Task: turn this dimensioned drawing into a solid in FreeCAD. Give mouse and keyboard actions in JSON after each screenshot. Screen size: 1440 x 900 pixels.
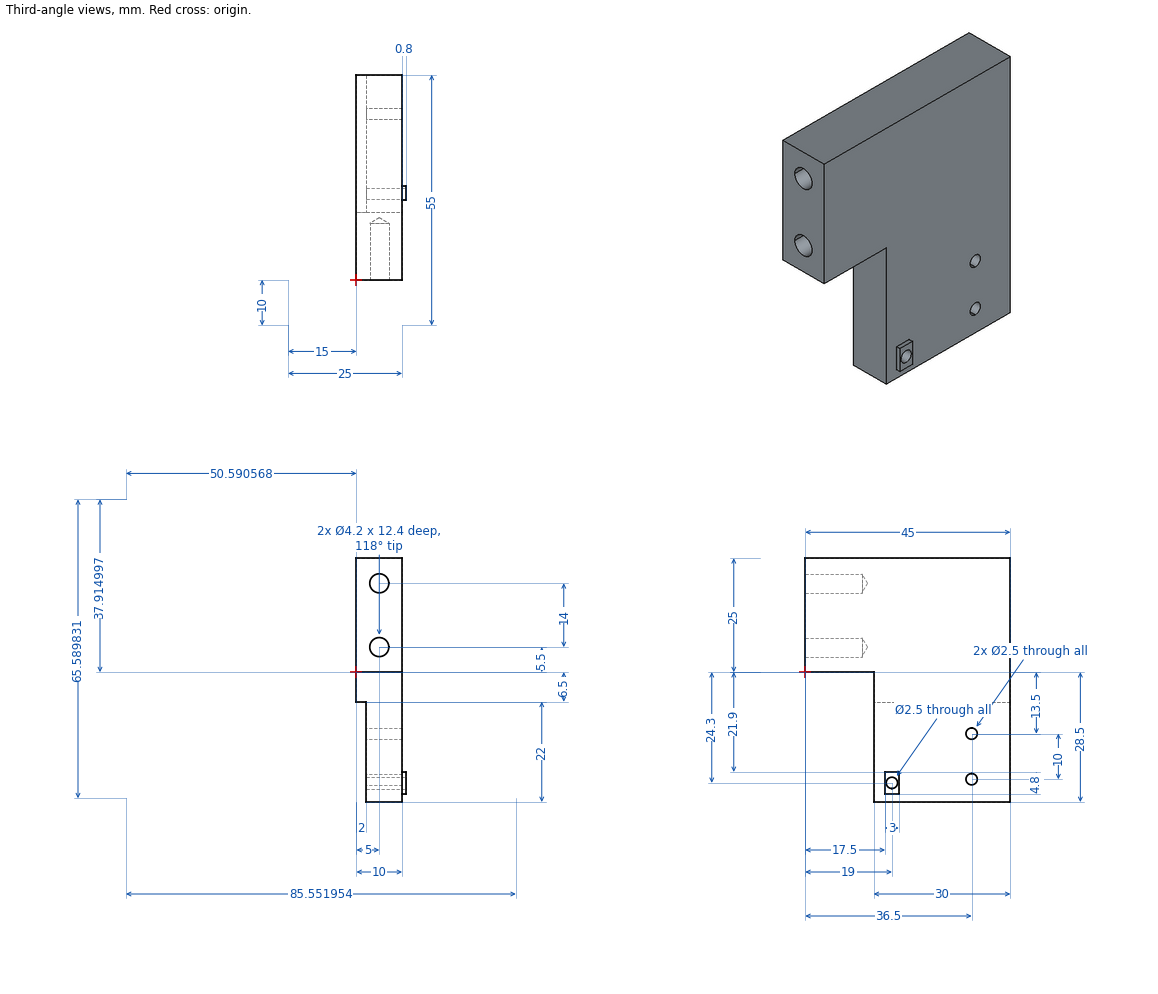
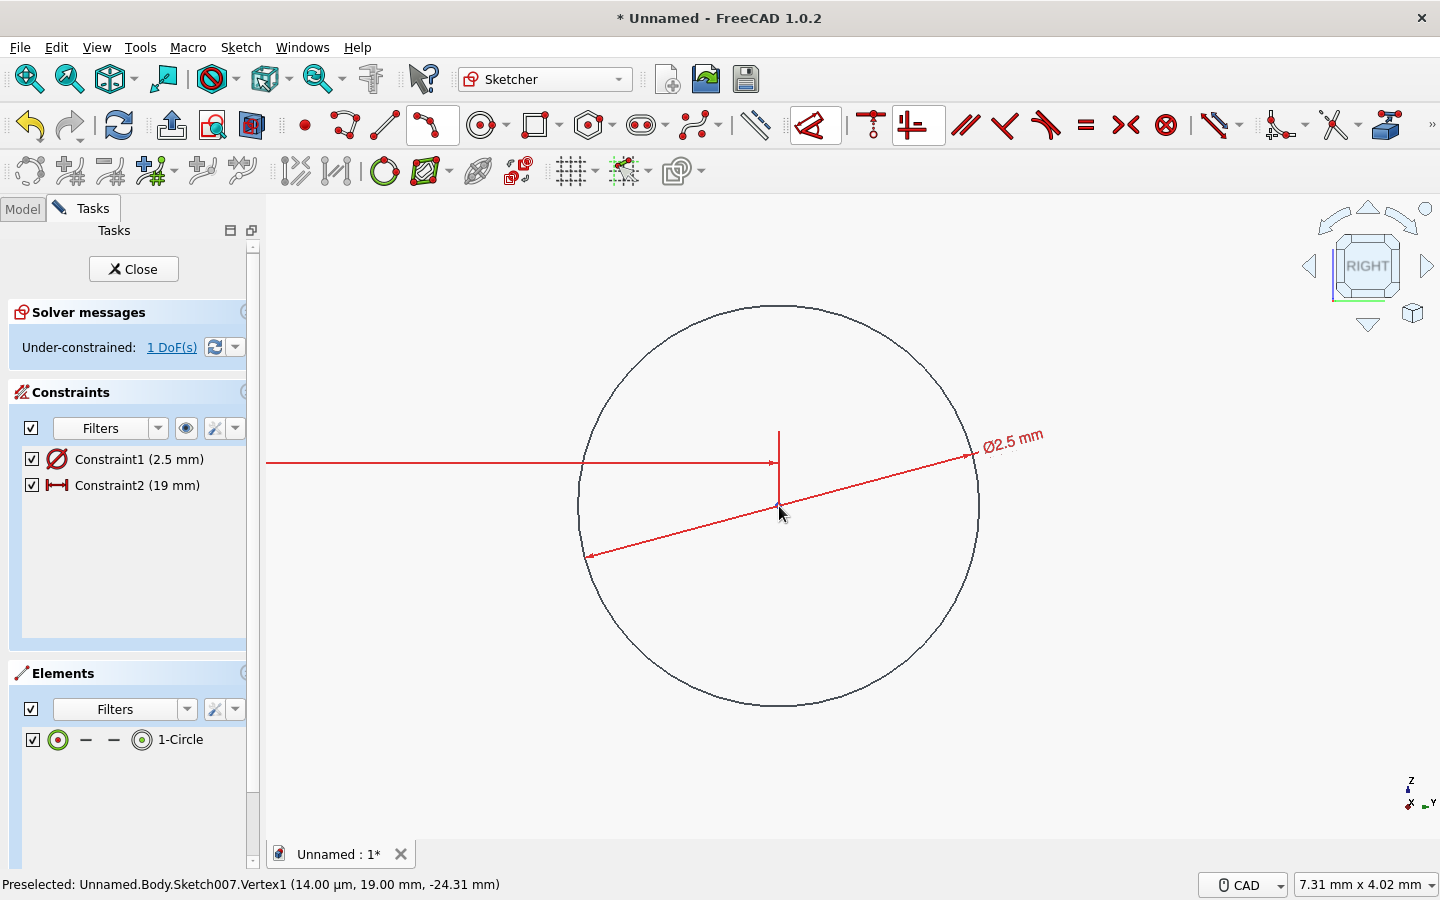
{"action": "left_click", "coordinate": [779, 506]}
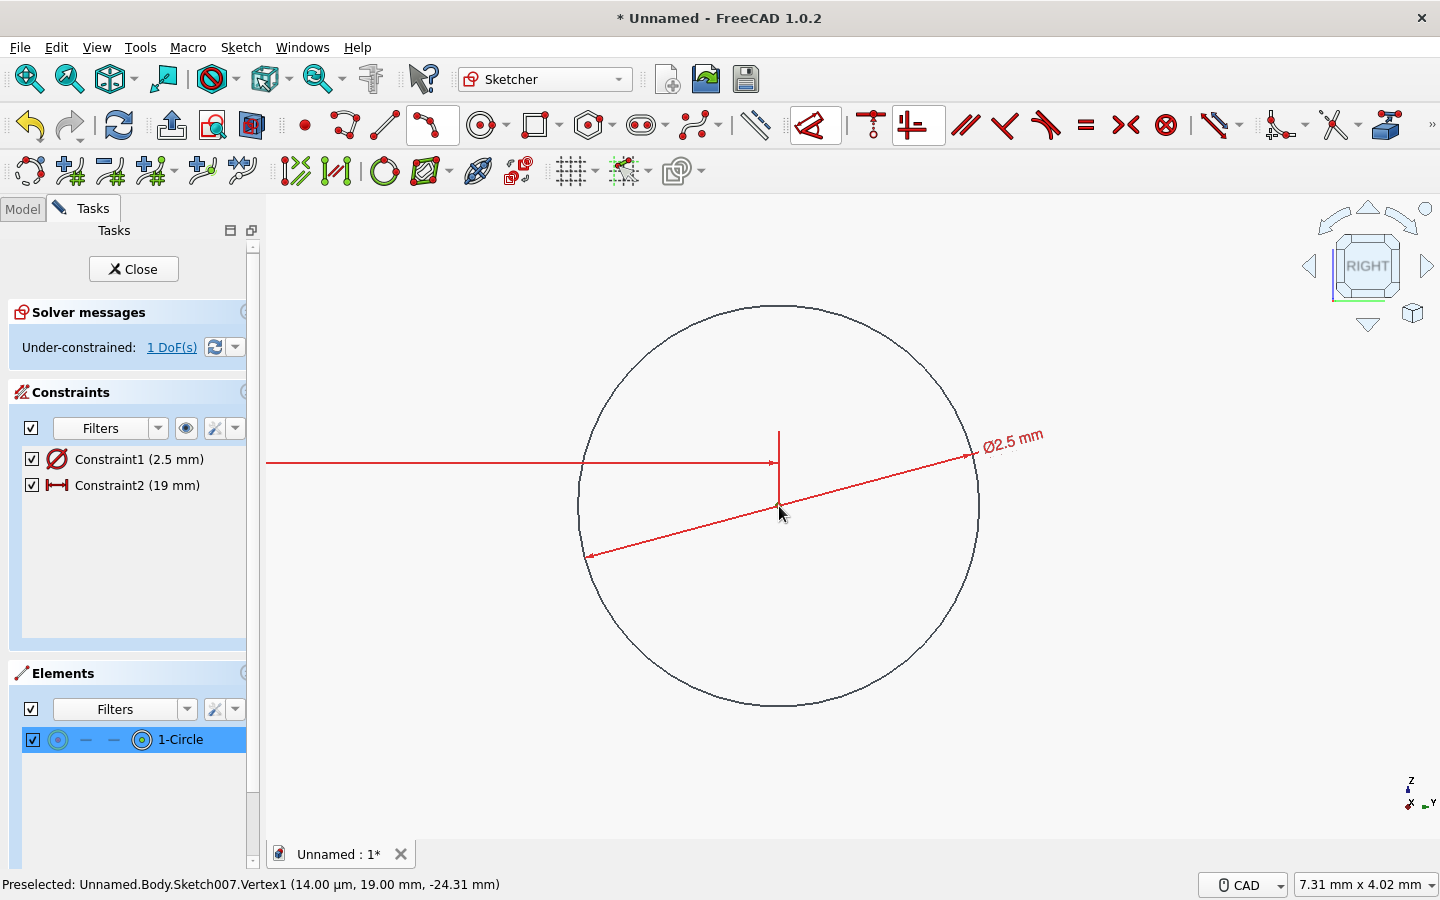
{"action": "left_click", "coordinate": [836, 126]}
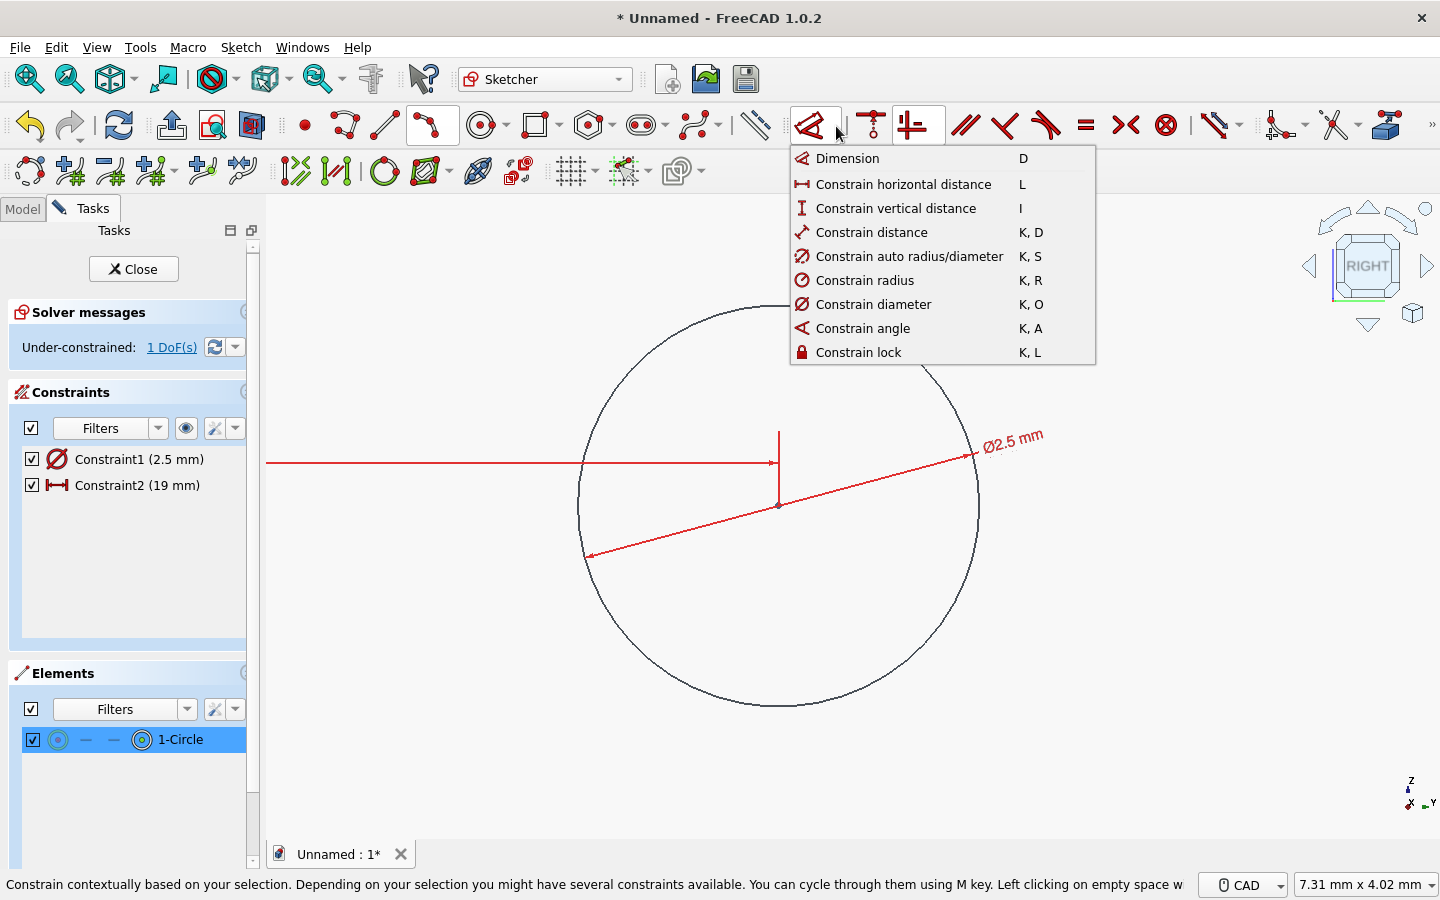
{"action": "left_click", "coordinate": [943, 208]}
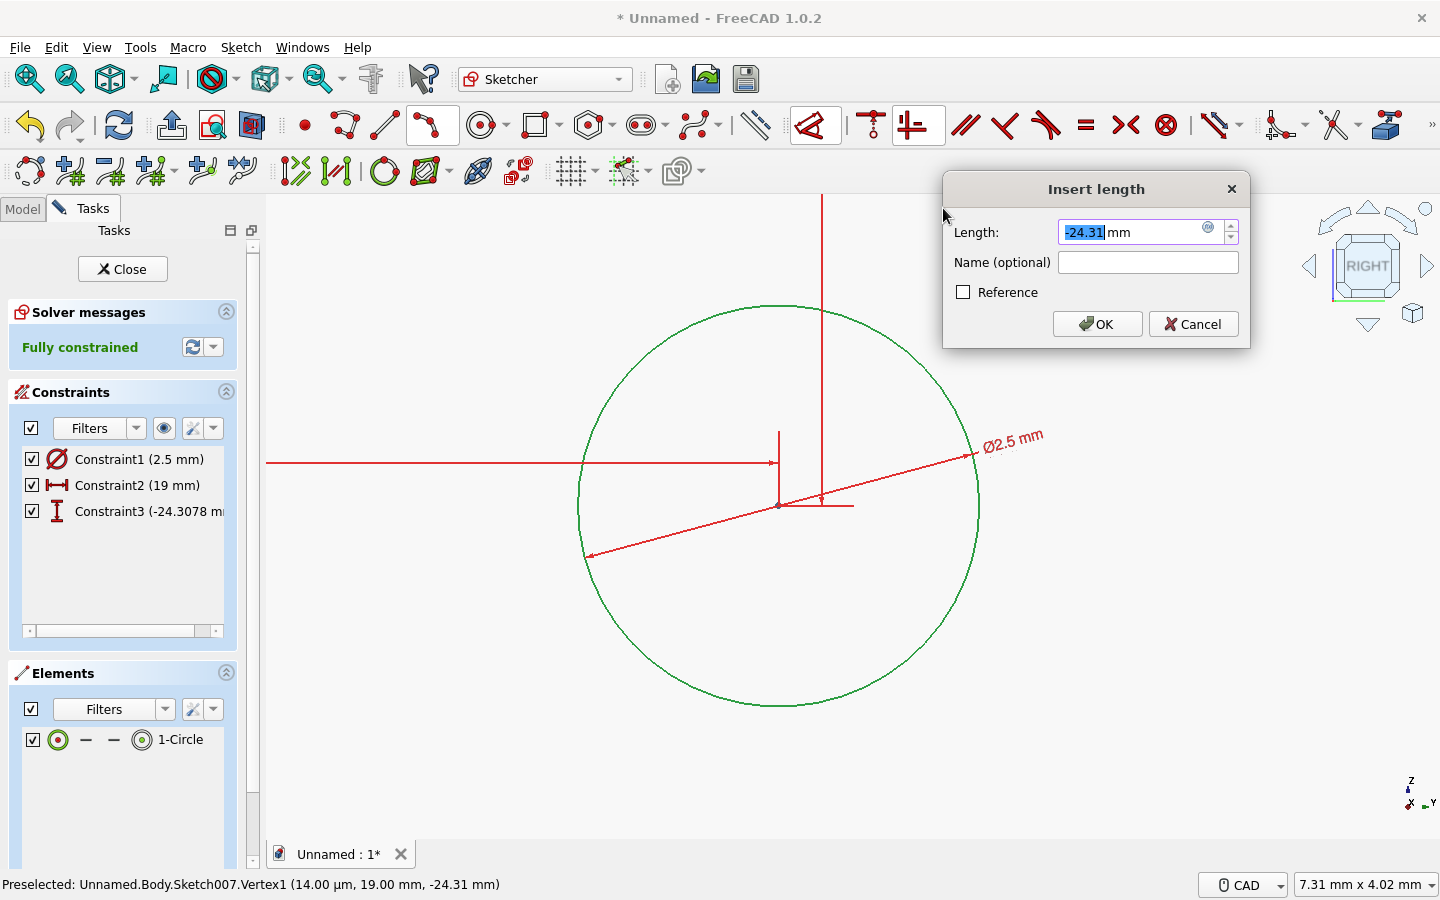
{"action": "type", "text": "-24.3"}
{"action": "key", "text": "Return"}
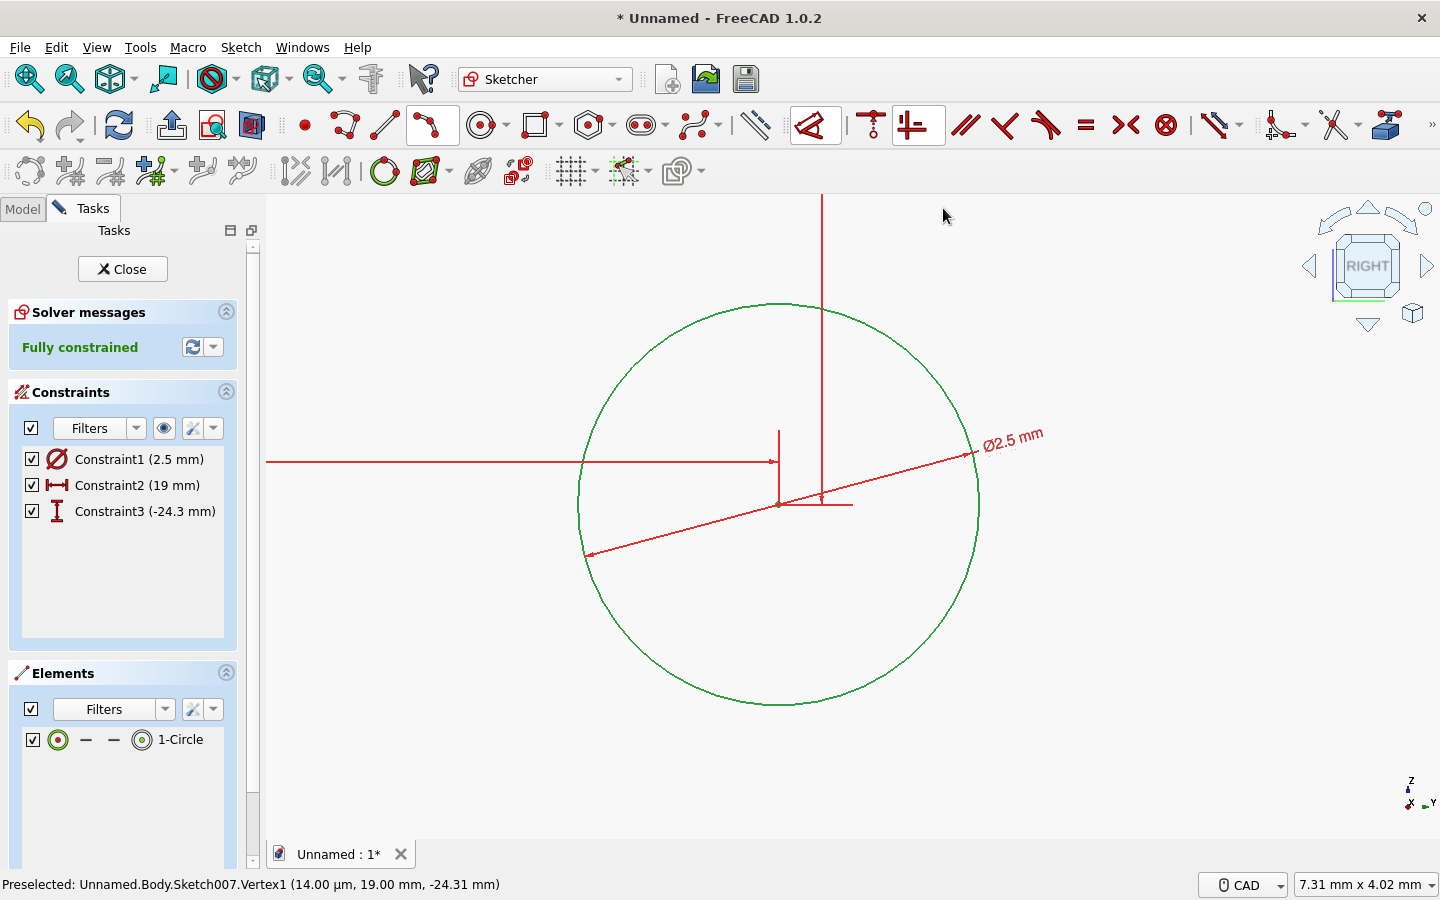
{"action": "left_click", "coordinate": [123, 269]}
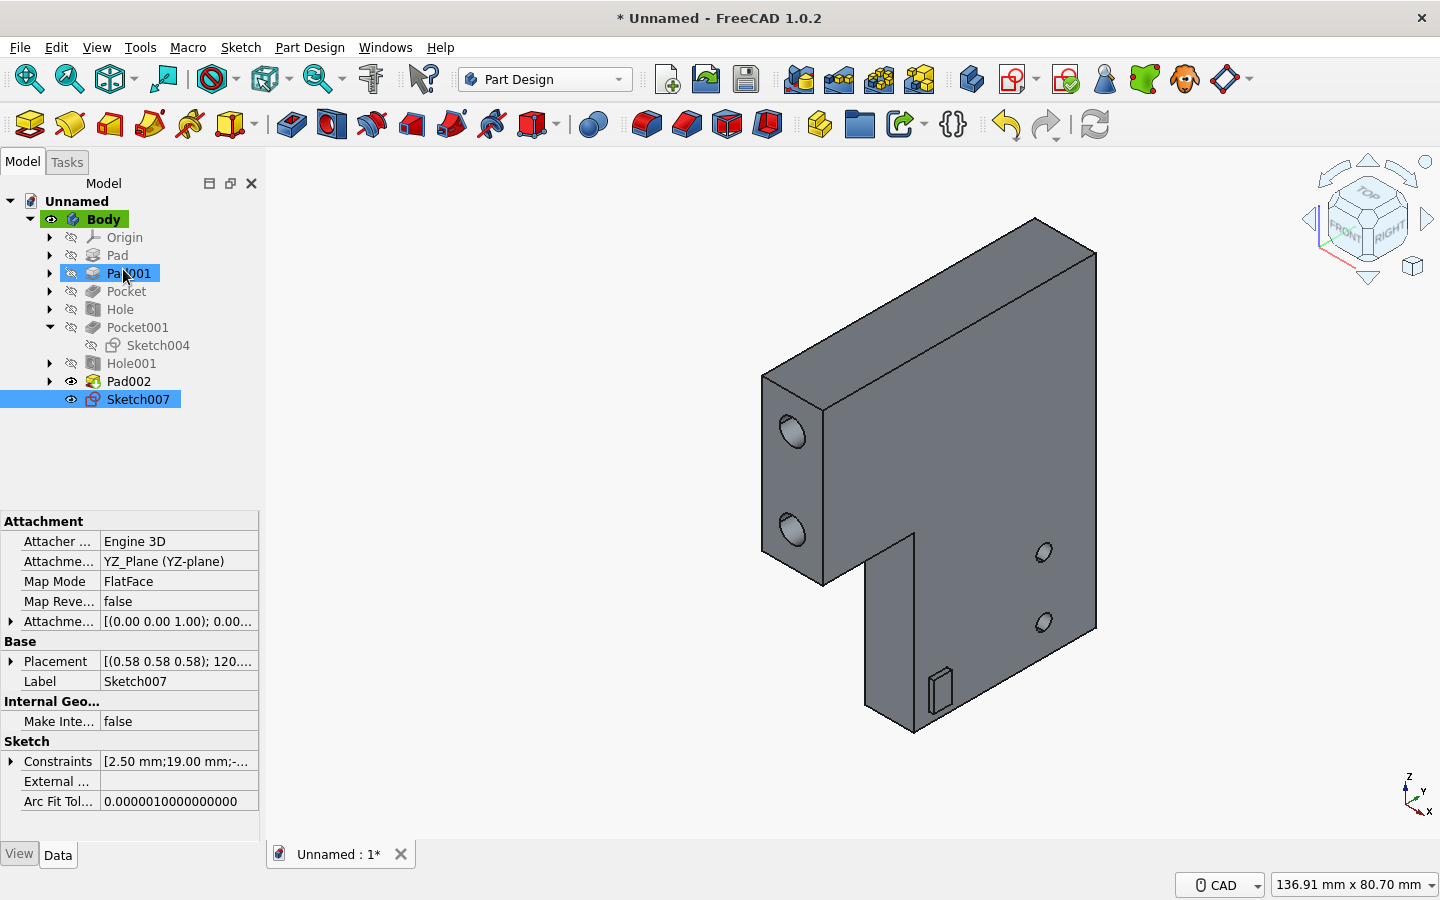
{"action": "left_click", "coordinate": [332, 124]}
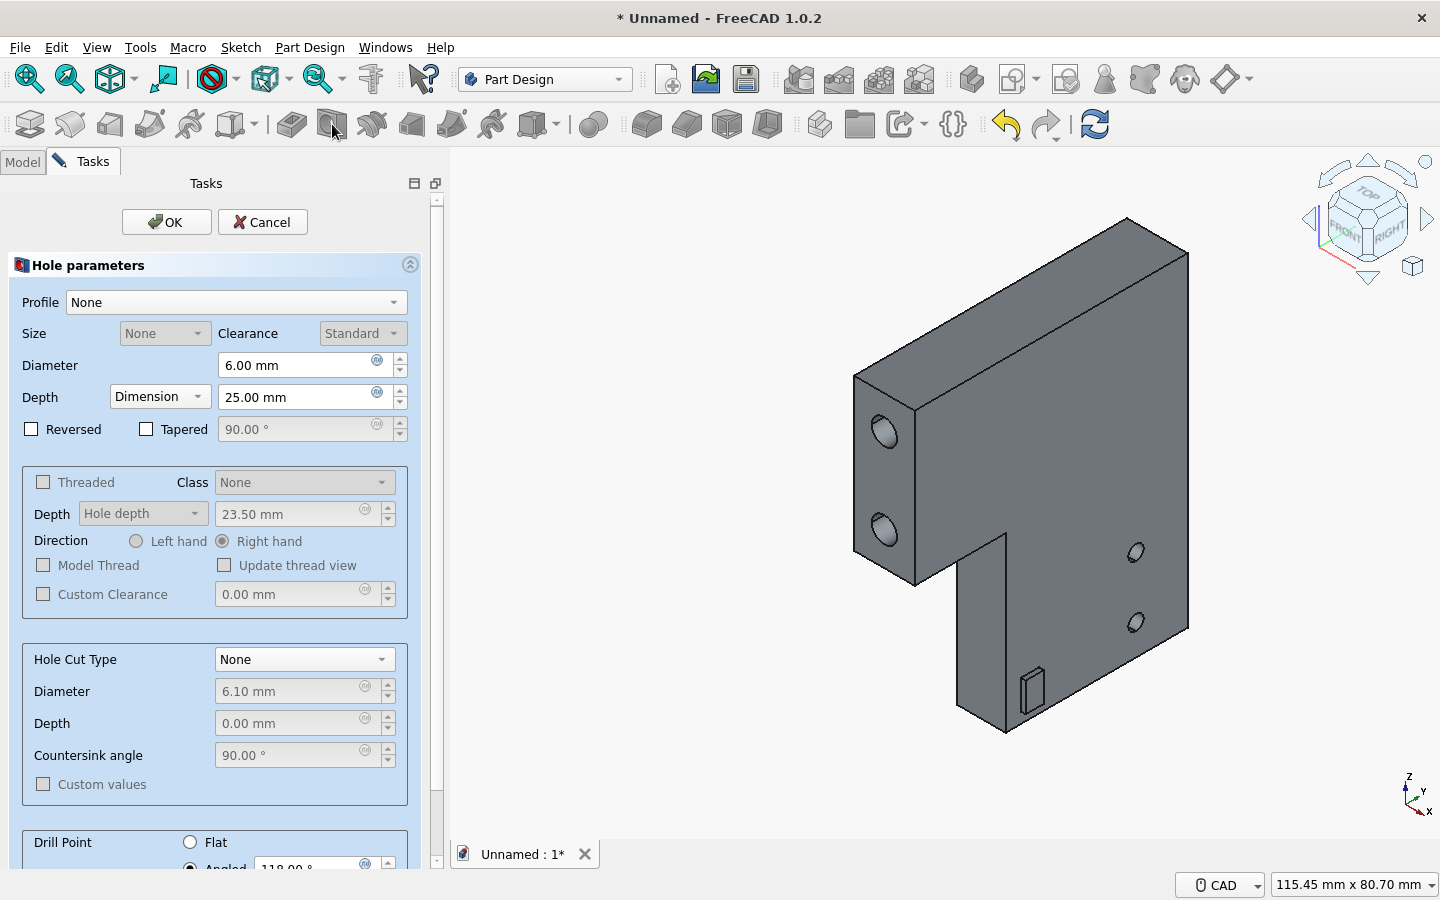
{"action": "triple_click", "coordinate": [305, 365]}